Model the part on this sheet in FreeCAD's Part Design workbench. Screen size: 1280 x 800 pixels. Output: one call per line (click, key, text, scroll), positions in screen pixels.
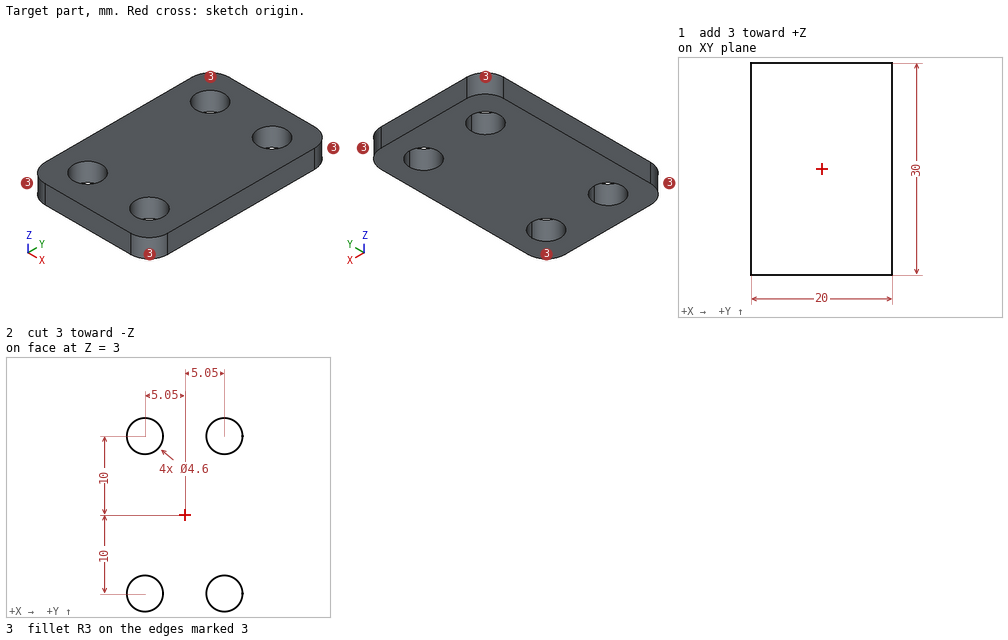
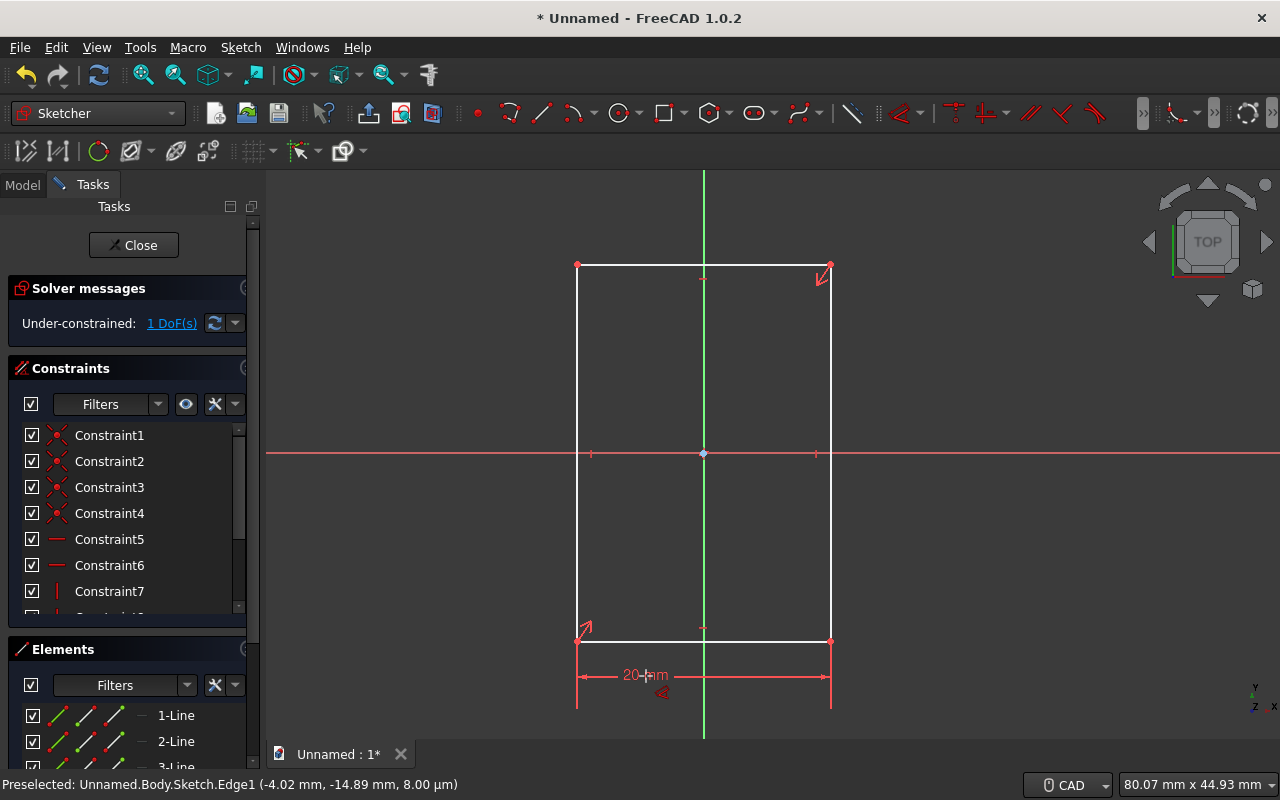
click(831, 529)
click(865, 367)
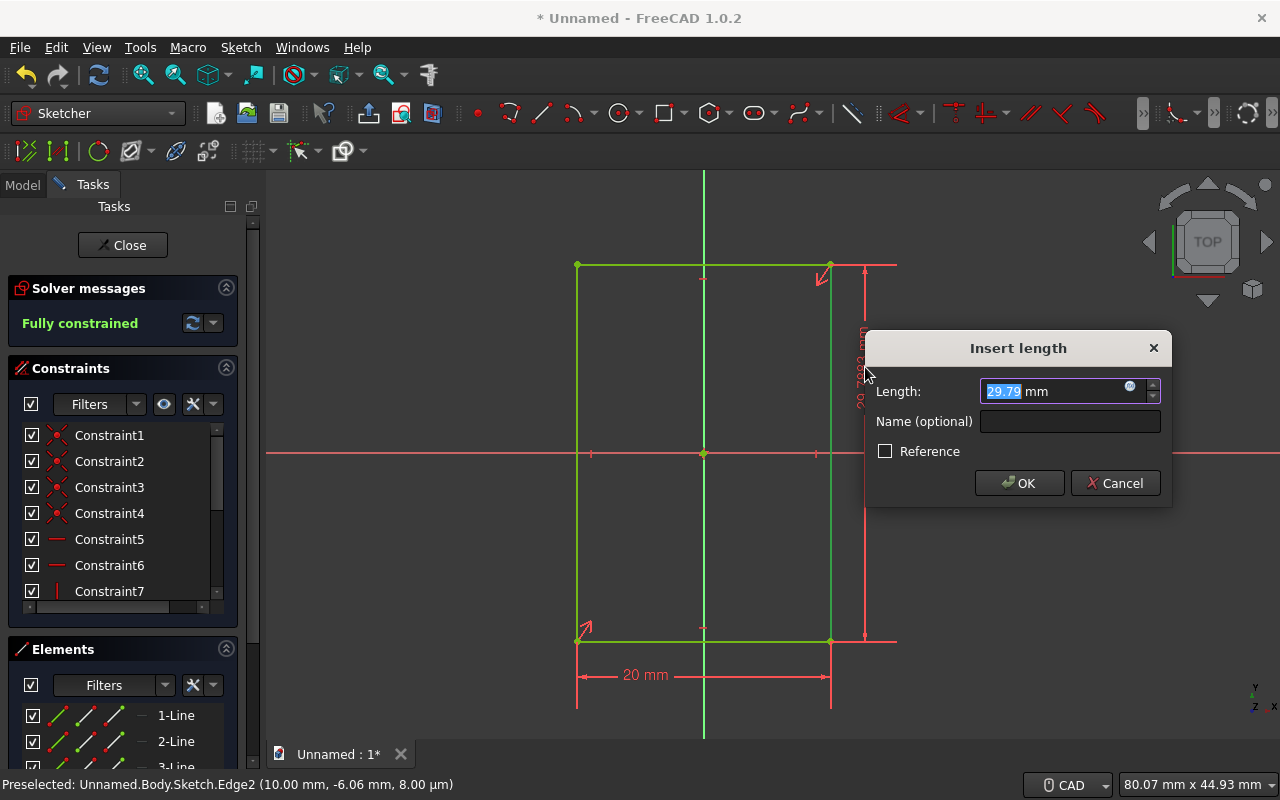
text(30)
key(Return)
key(Escape)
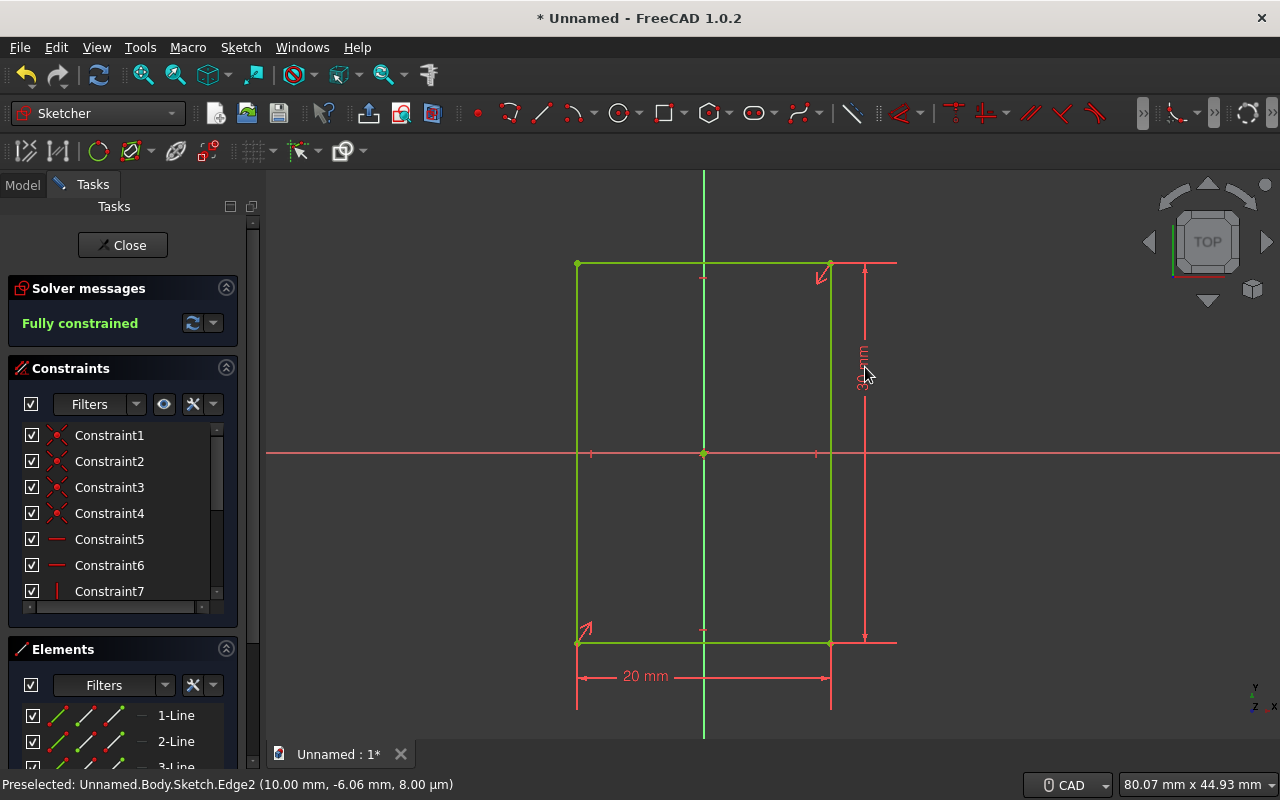
click(123, 245)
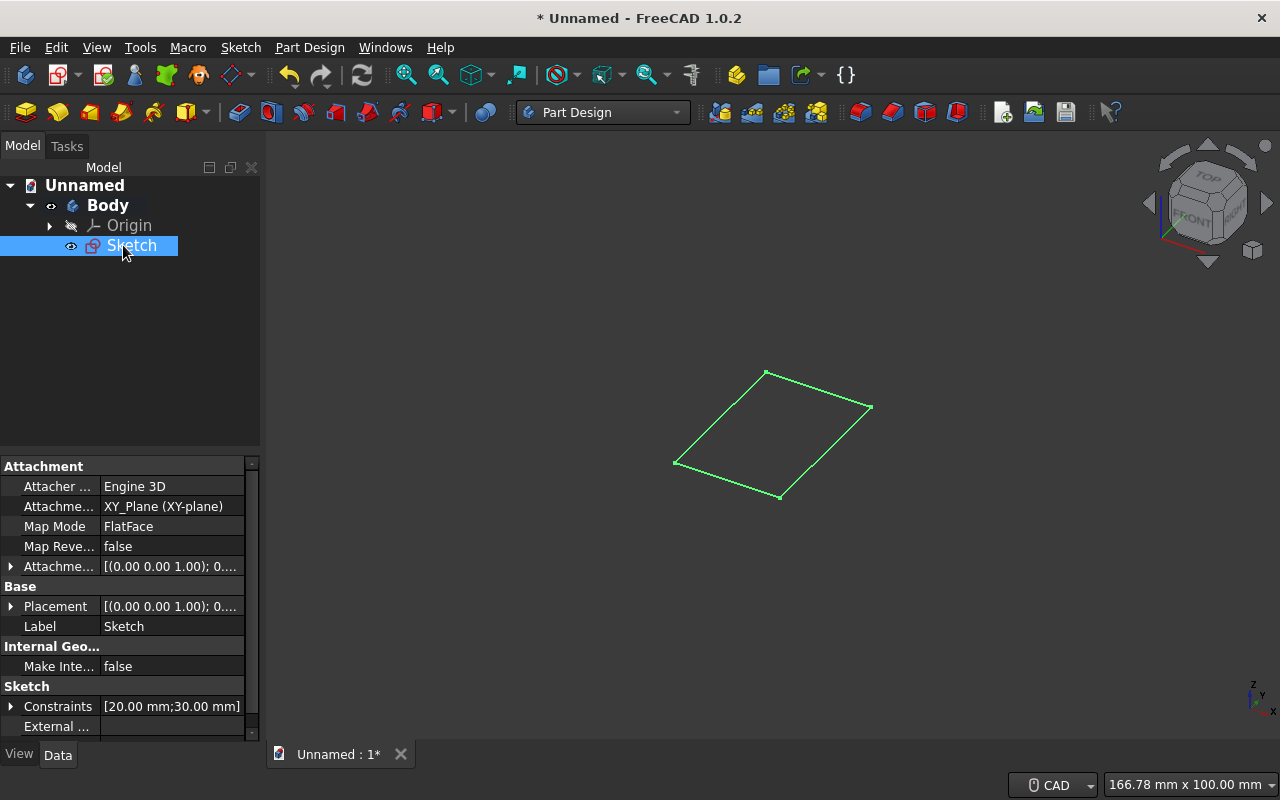
click(26, 112)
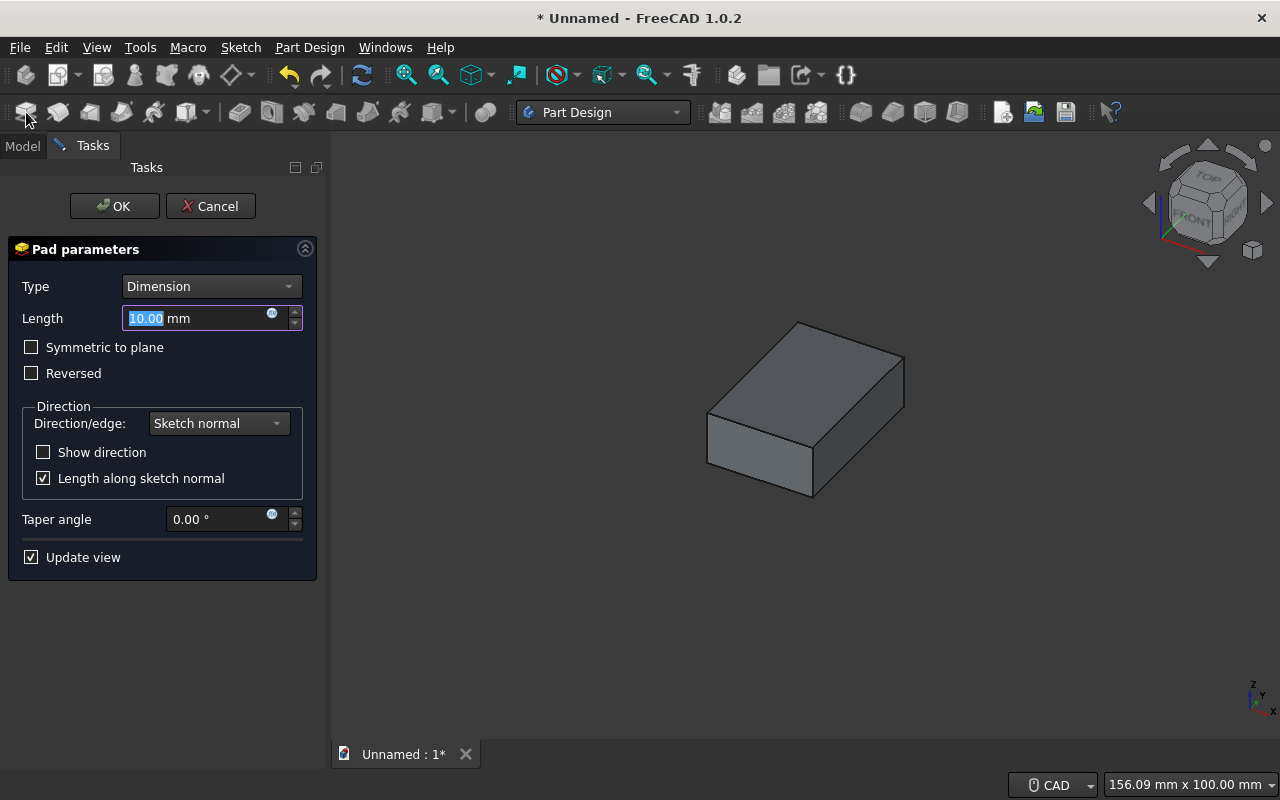
text(3)
key(Tab)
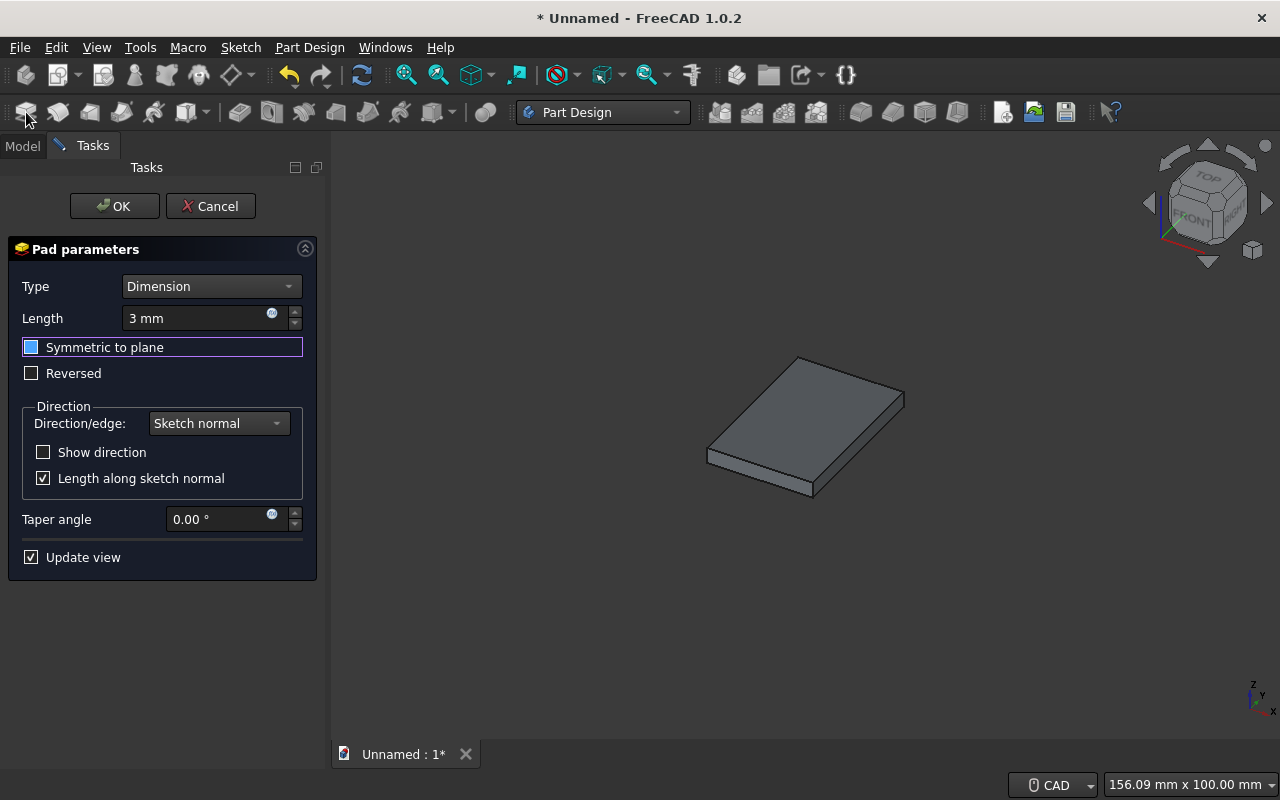
click(115, 206)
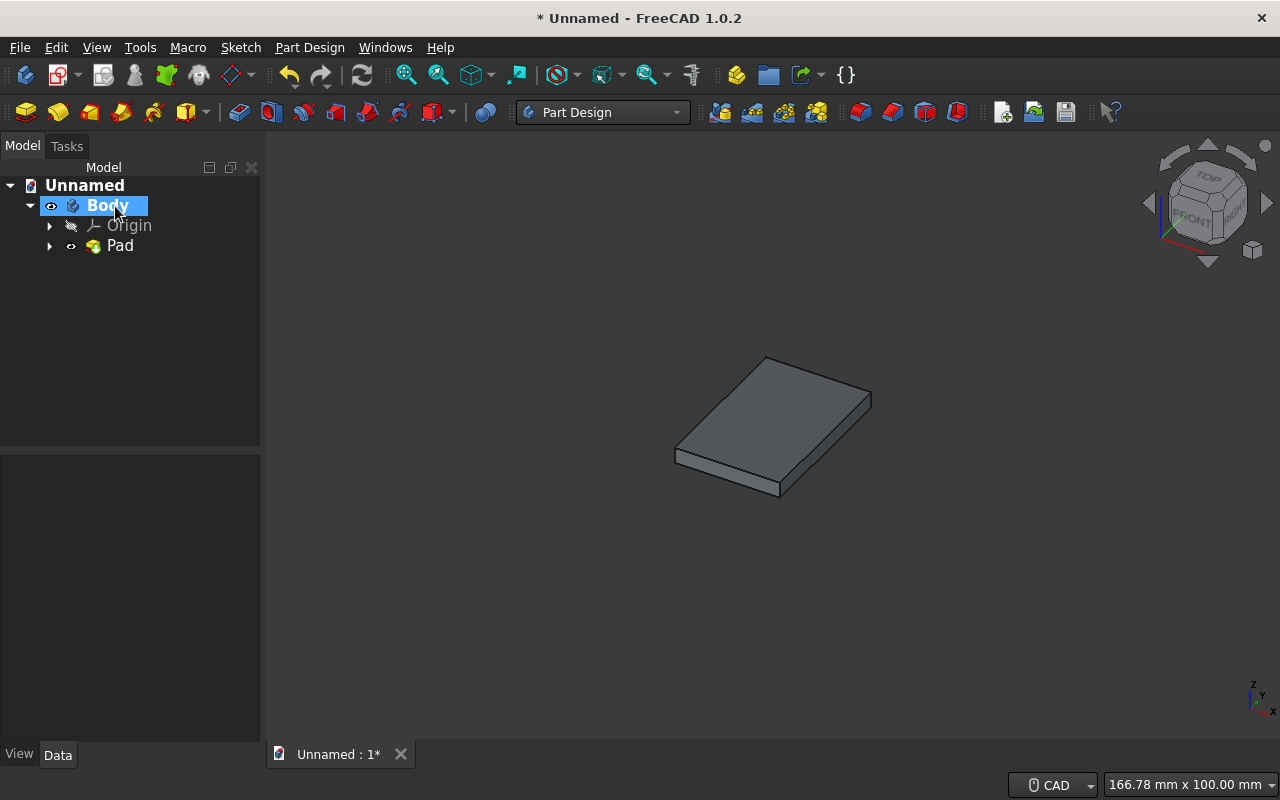
key(v)
key(f)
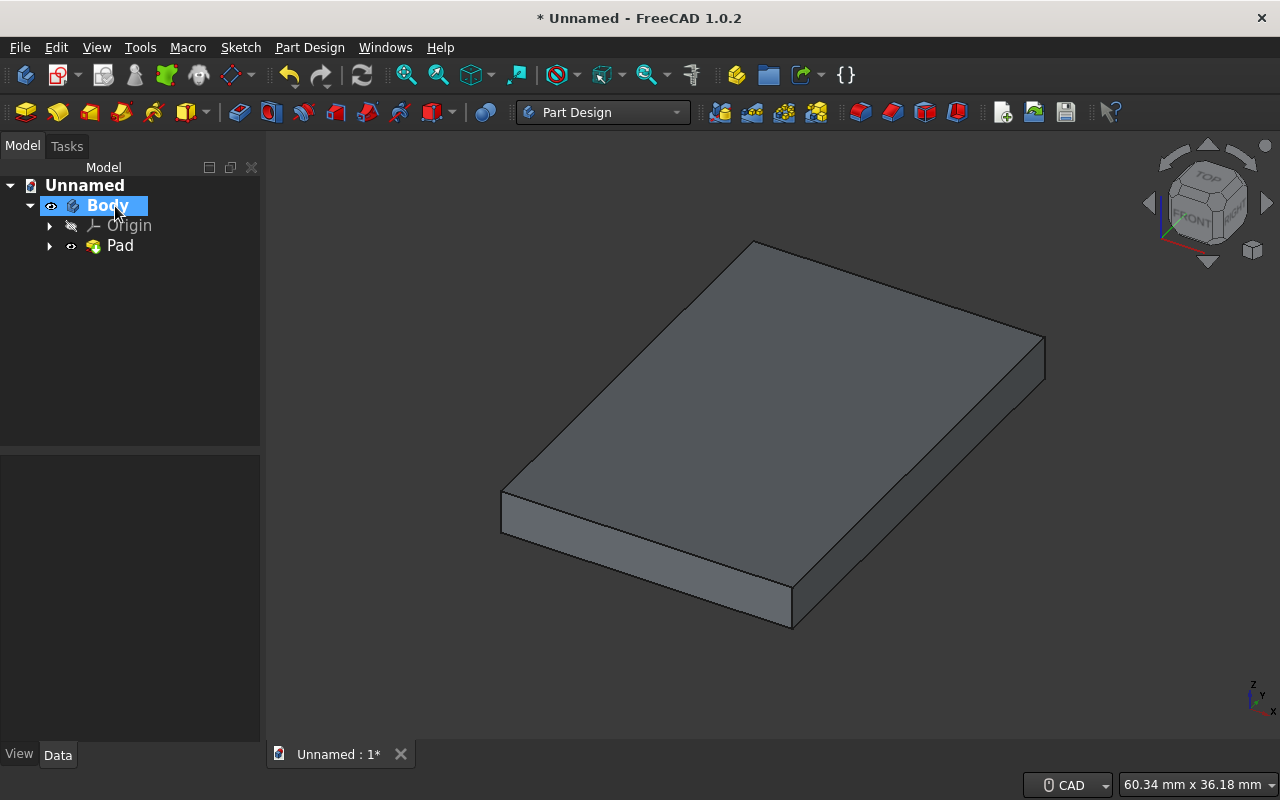
click(809, 378)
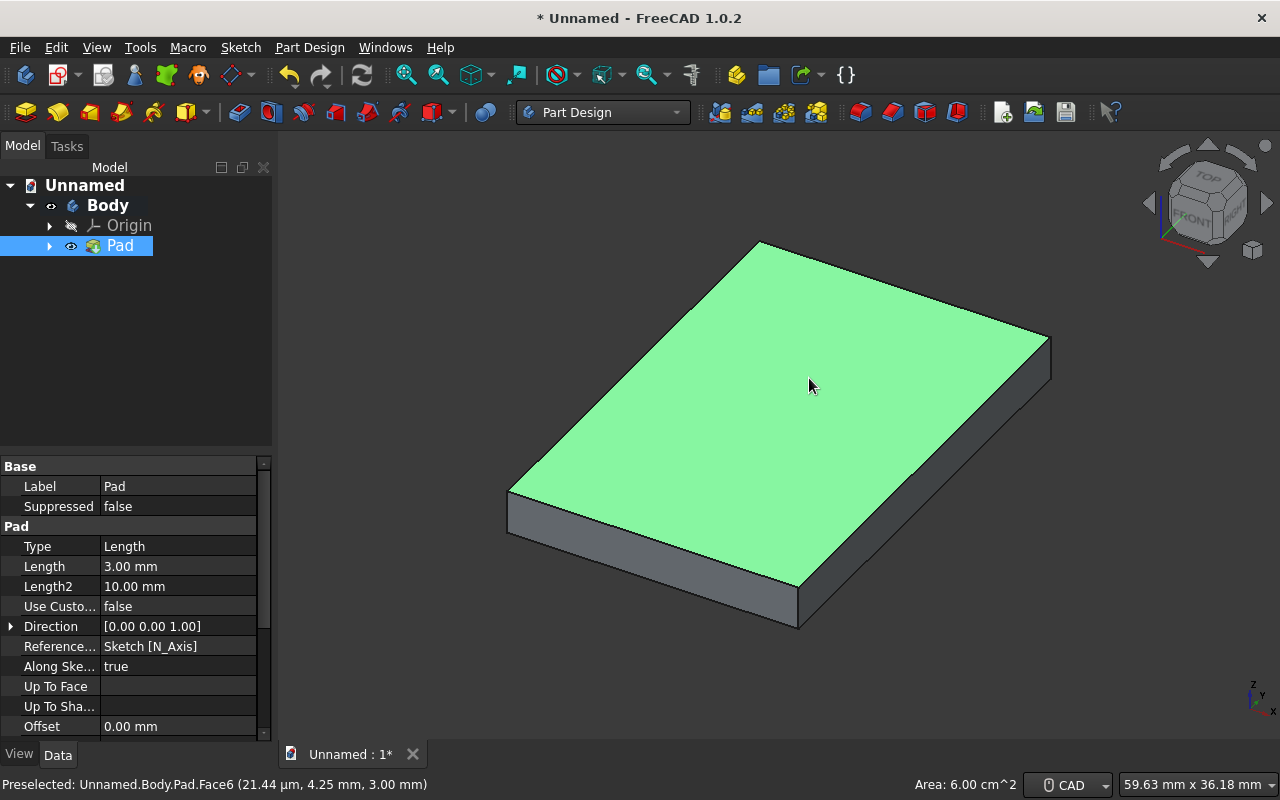
click(58, 76)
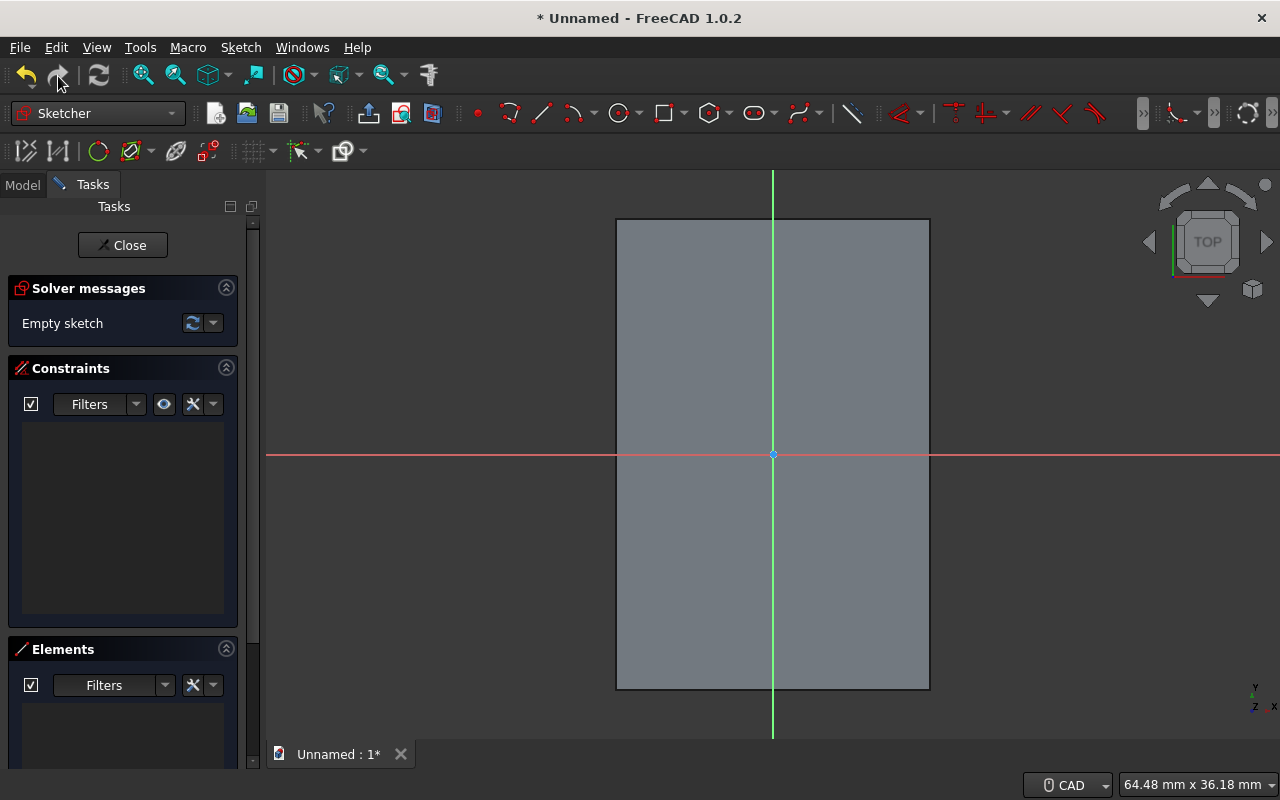
click(620, 114)